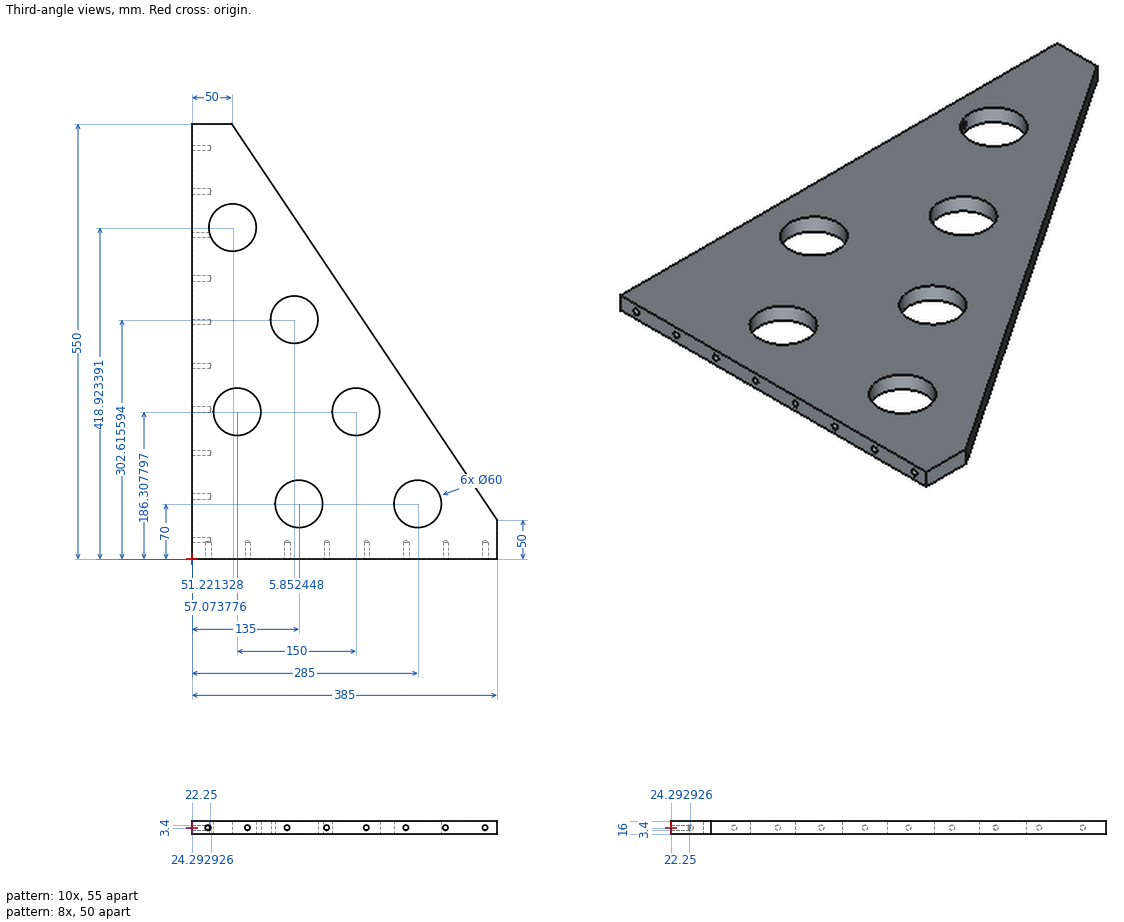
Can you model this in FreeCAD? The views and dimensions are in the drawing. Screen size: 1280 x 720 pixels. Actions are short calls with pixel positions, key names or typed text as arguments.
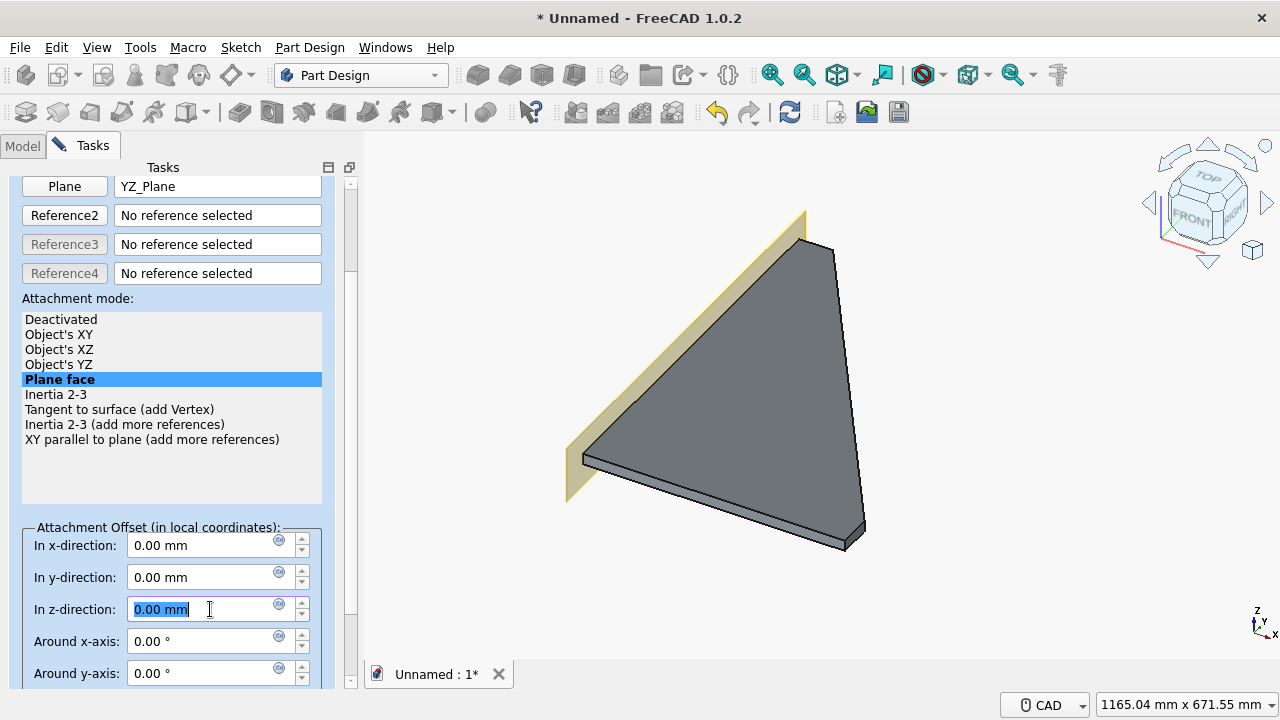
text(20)
key(Tab)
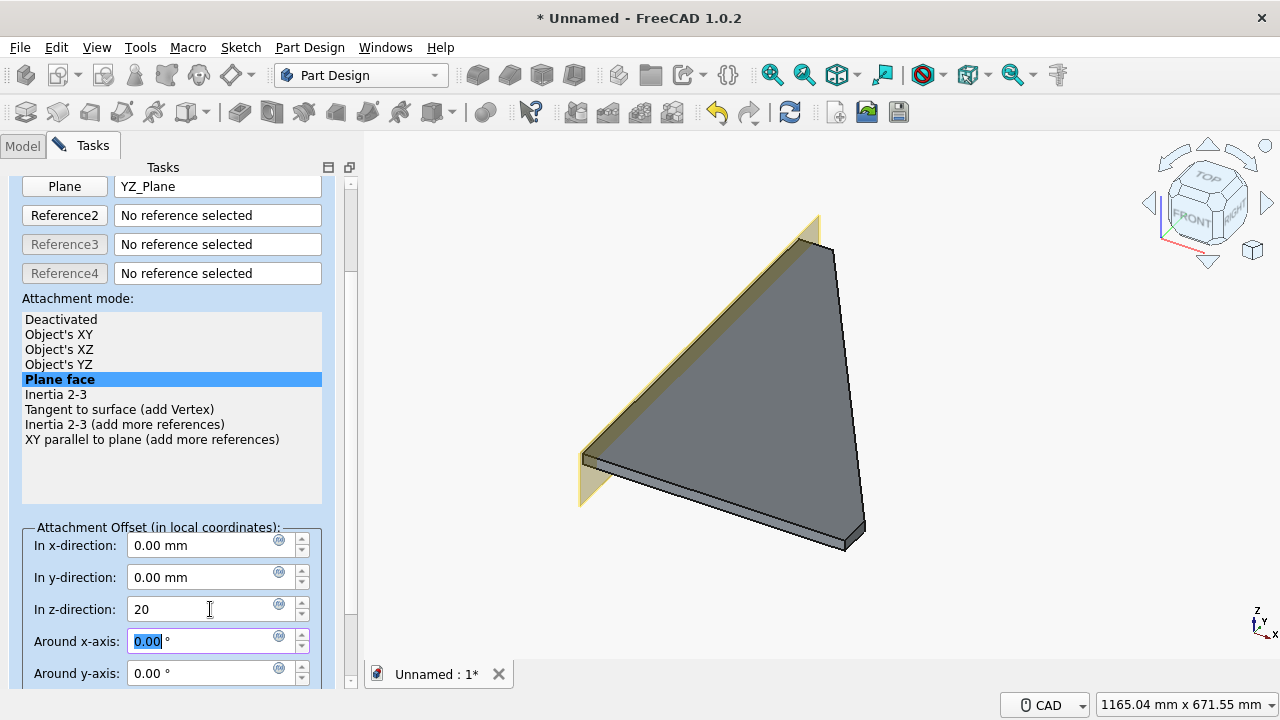
scroll(351, 432, up, 3)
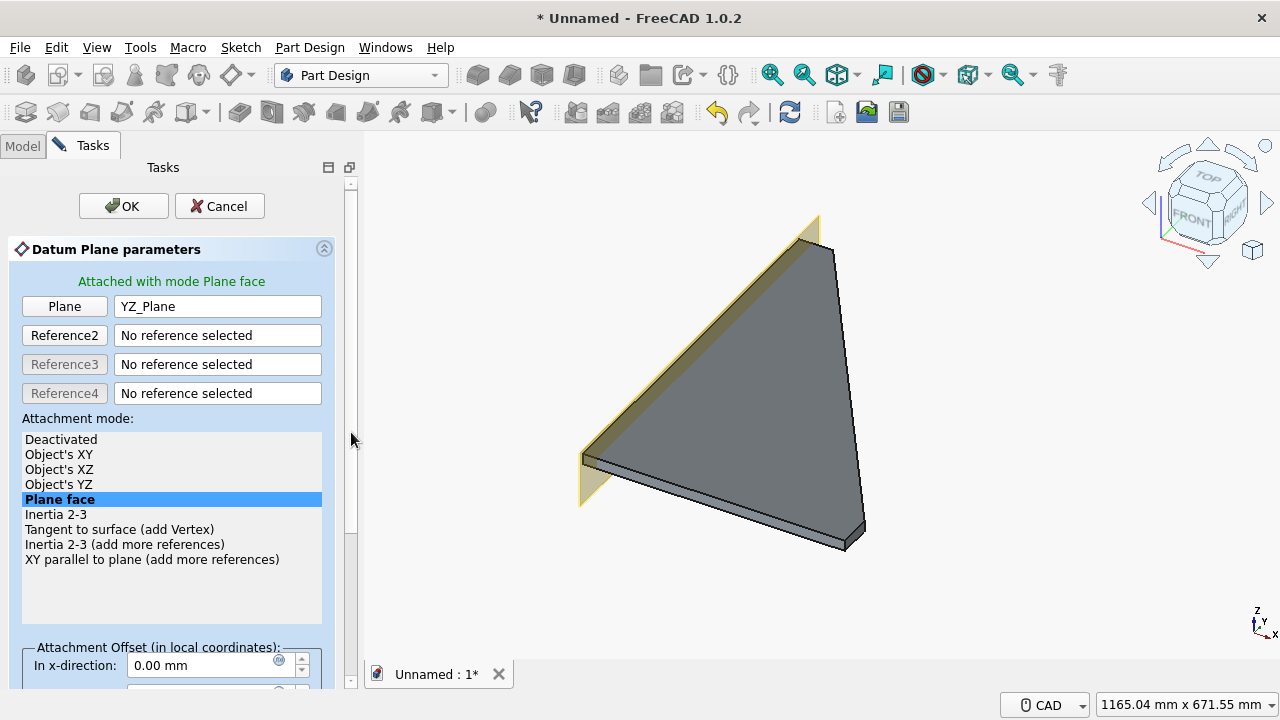
click(124, 206)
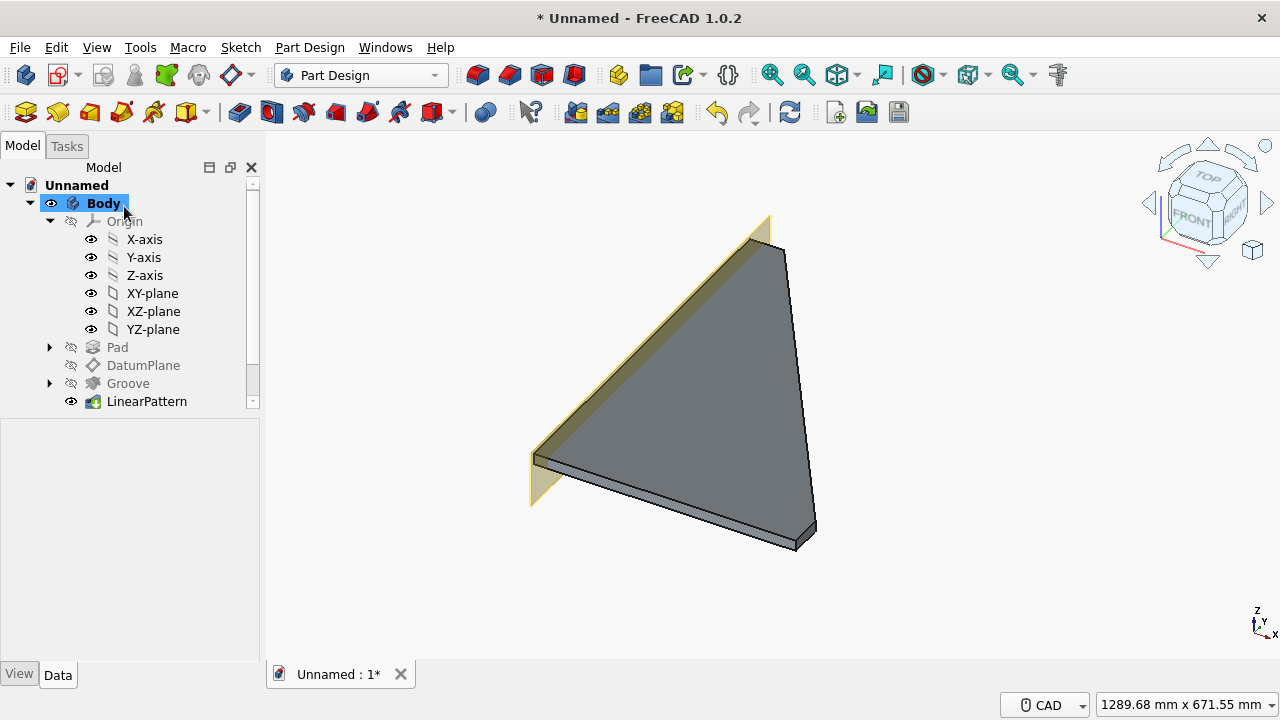
scroll(100, 289, down, 3)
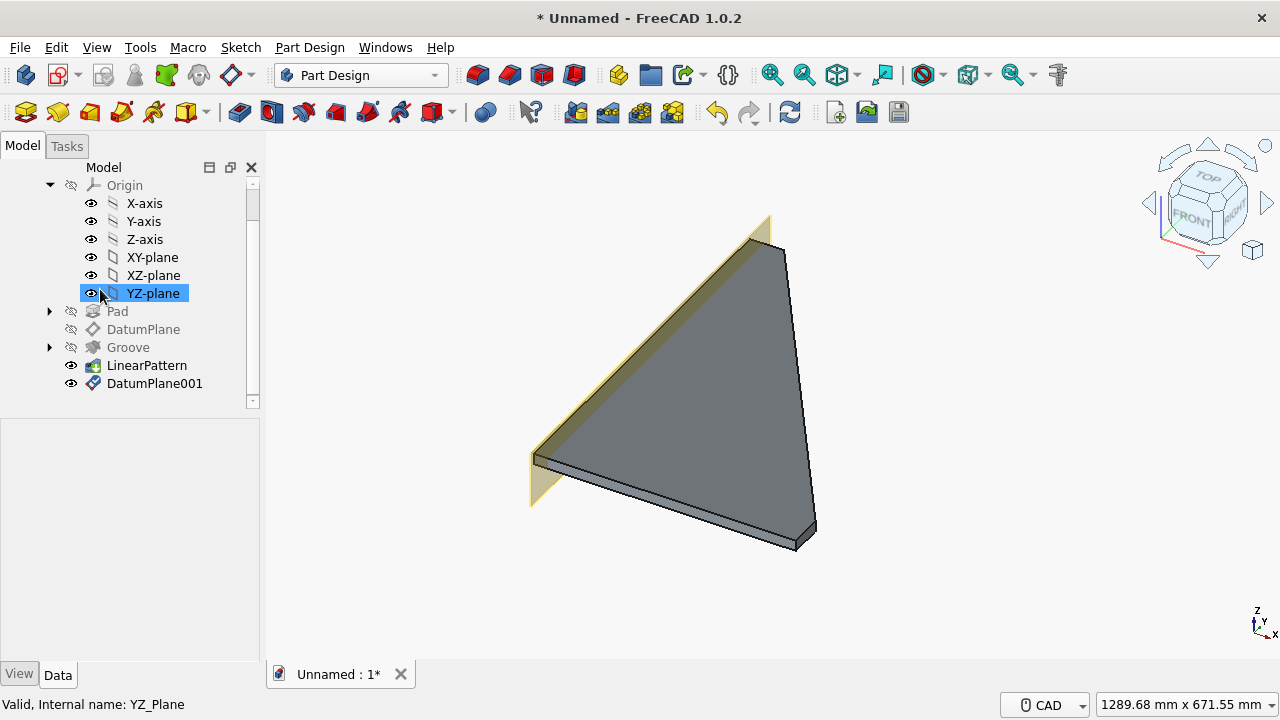
click(116, 383)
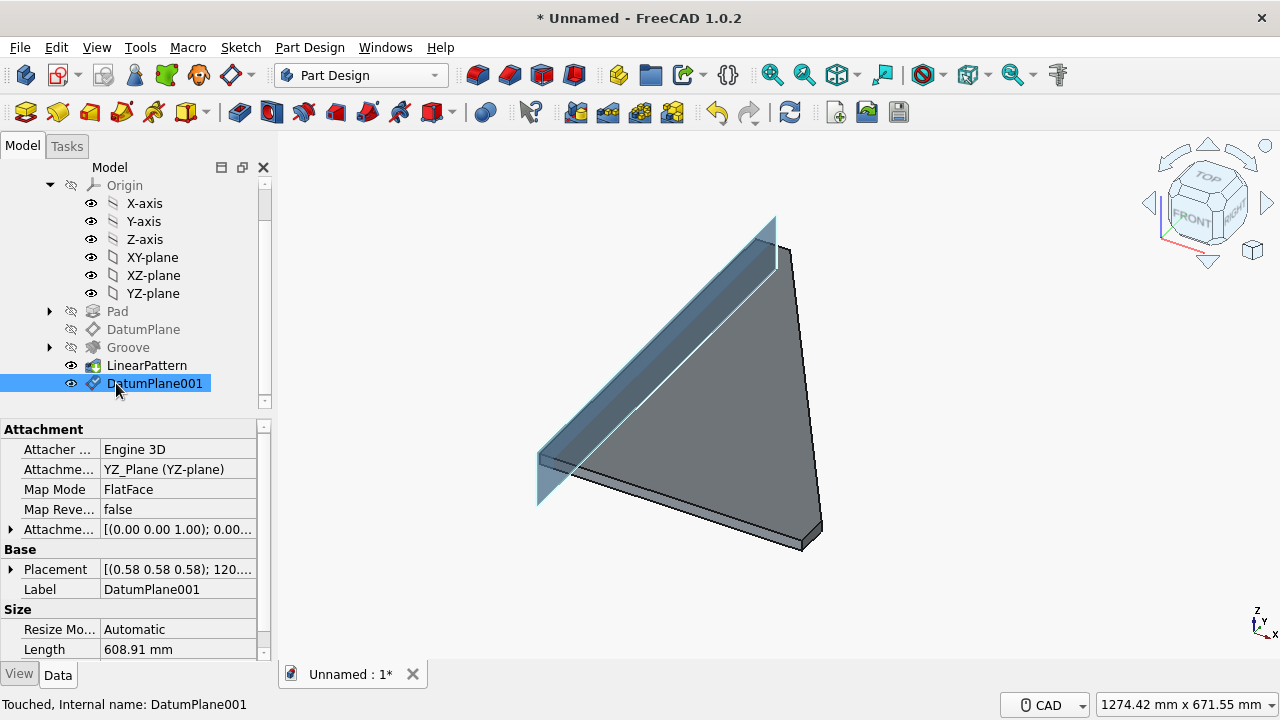
click(58, 76)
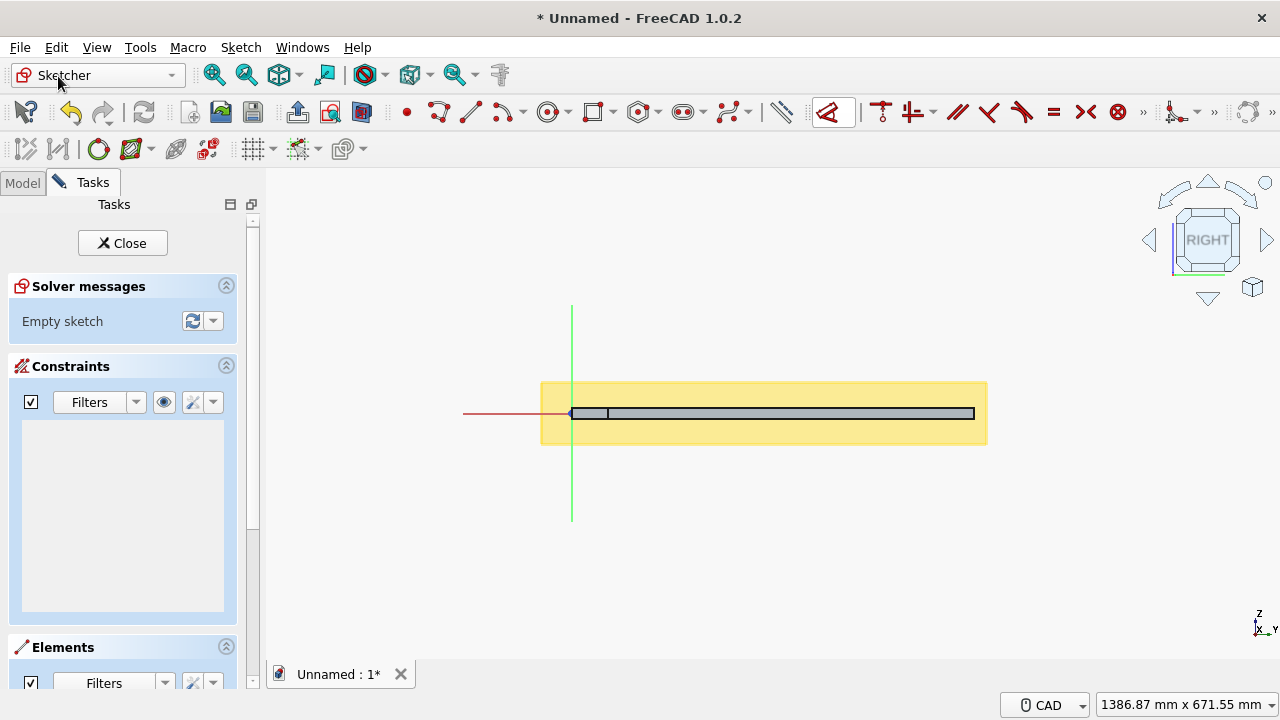
click(362, 112)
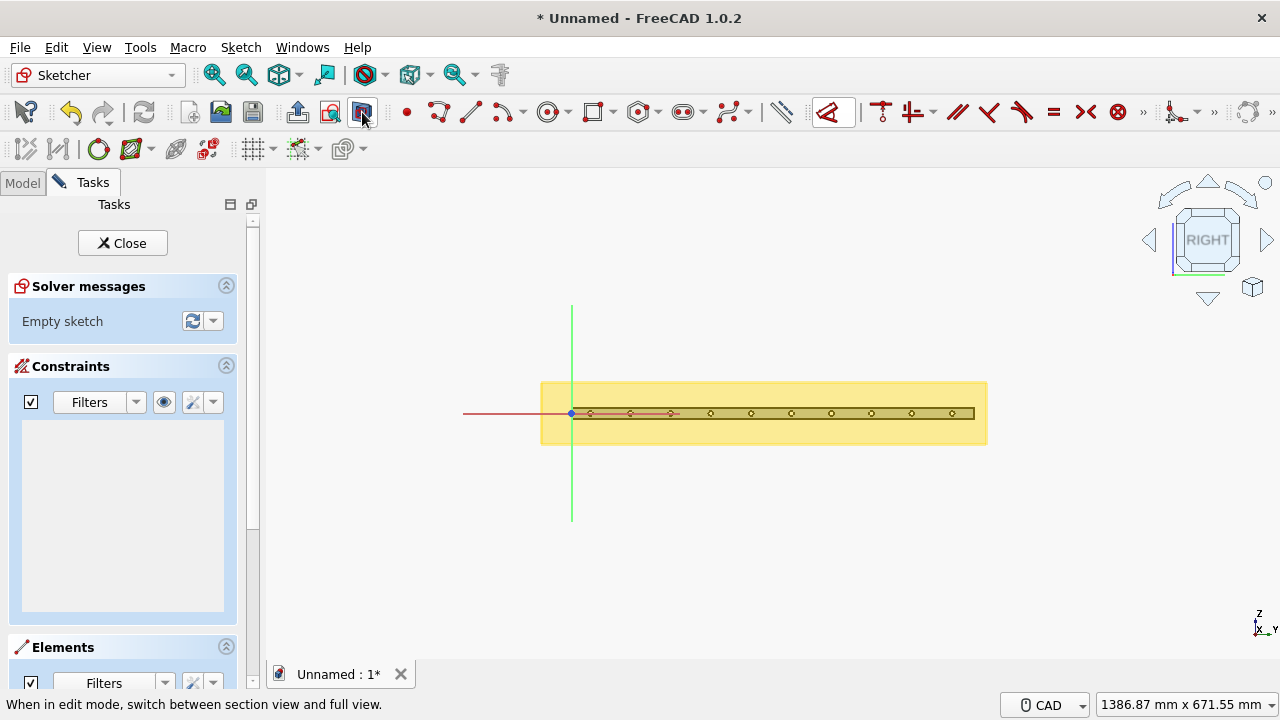
scroll(574, 415, up, 15)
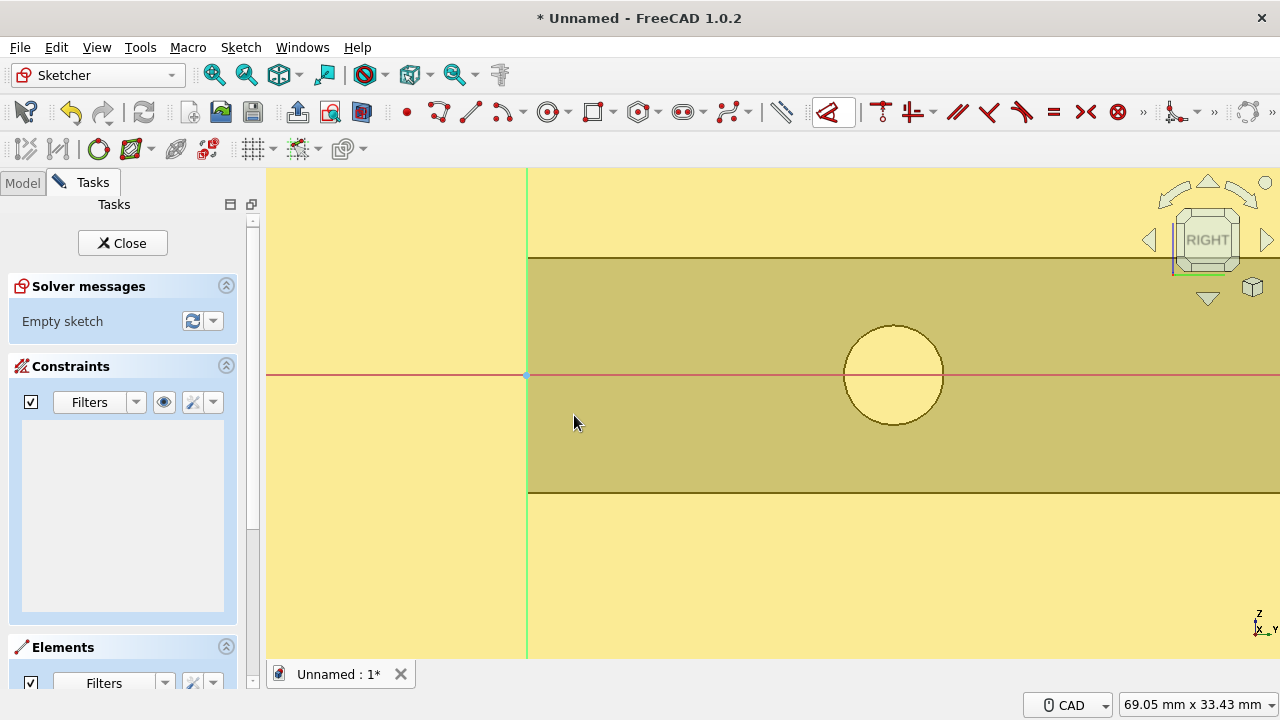
scroll(706, 373, up, 2)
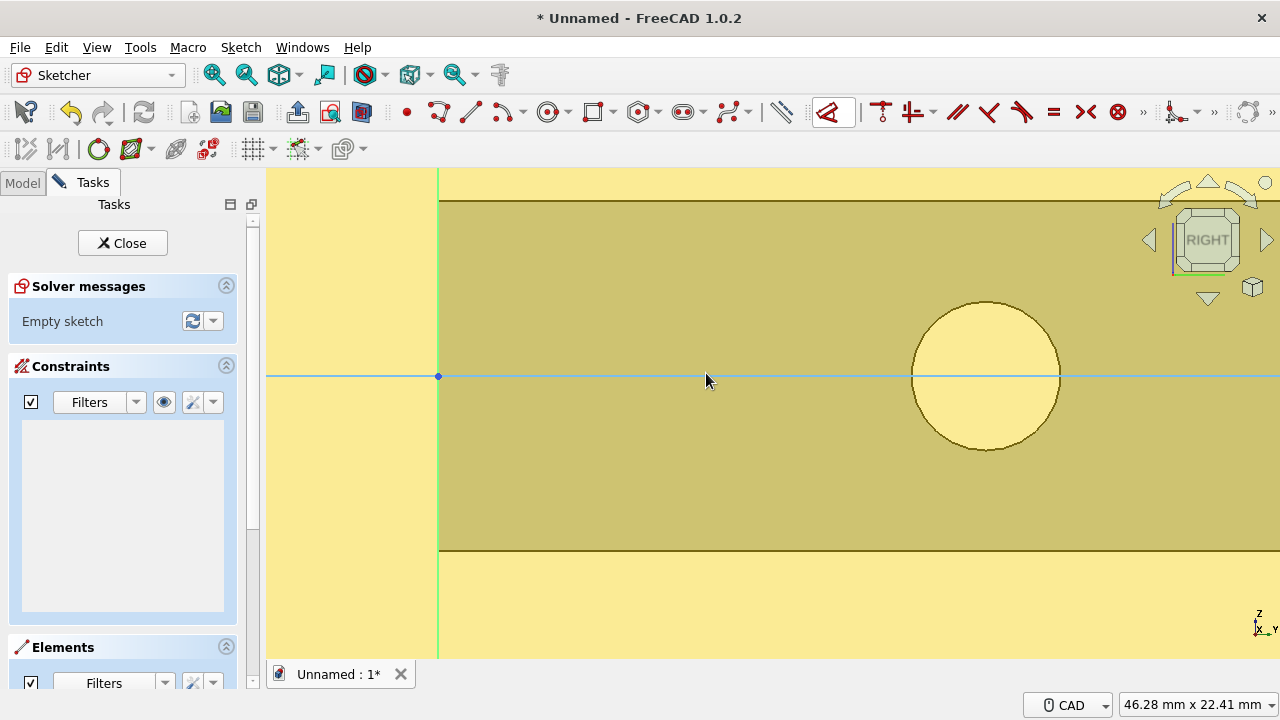
click(440, 112)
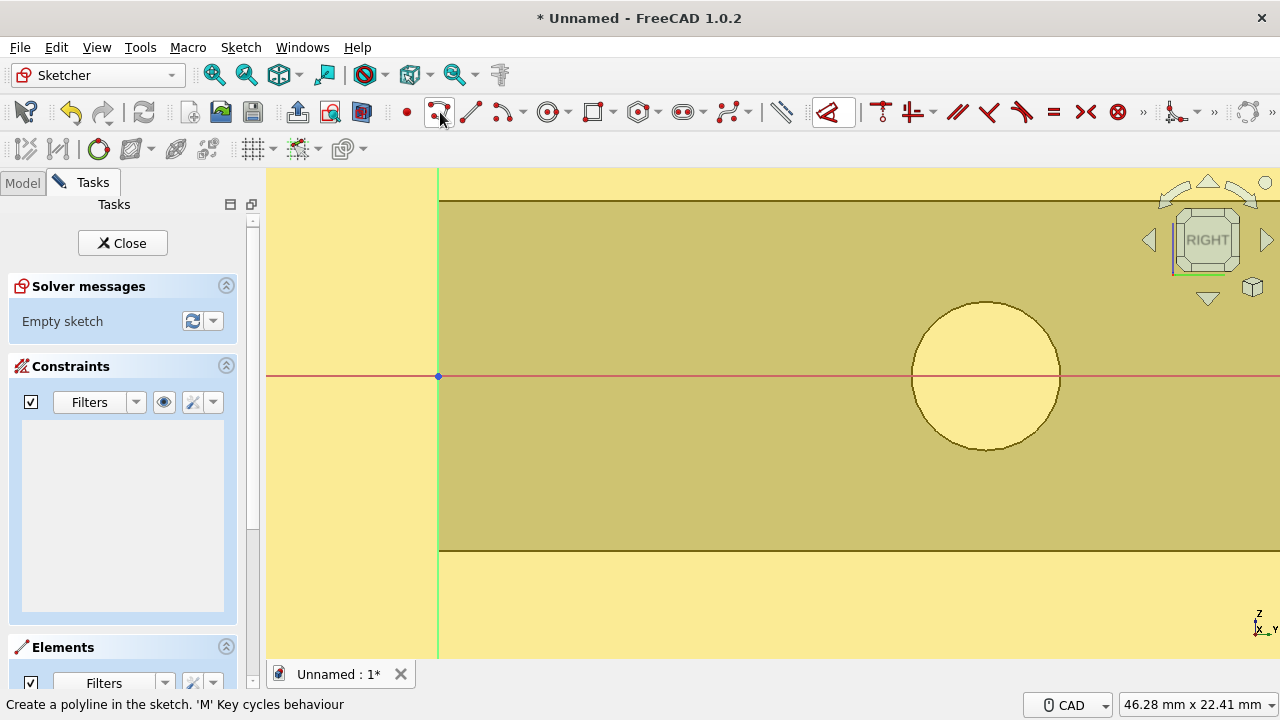
click(438, 376)
click(447, 451)
click(926, 451)
click(971, 385)
click(438, 376)
key(Escape)
key(Escape)